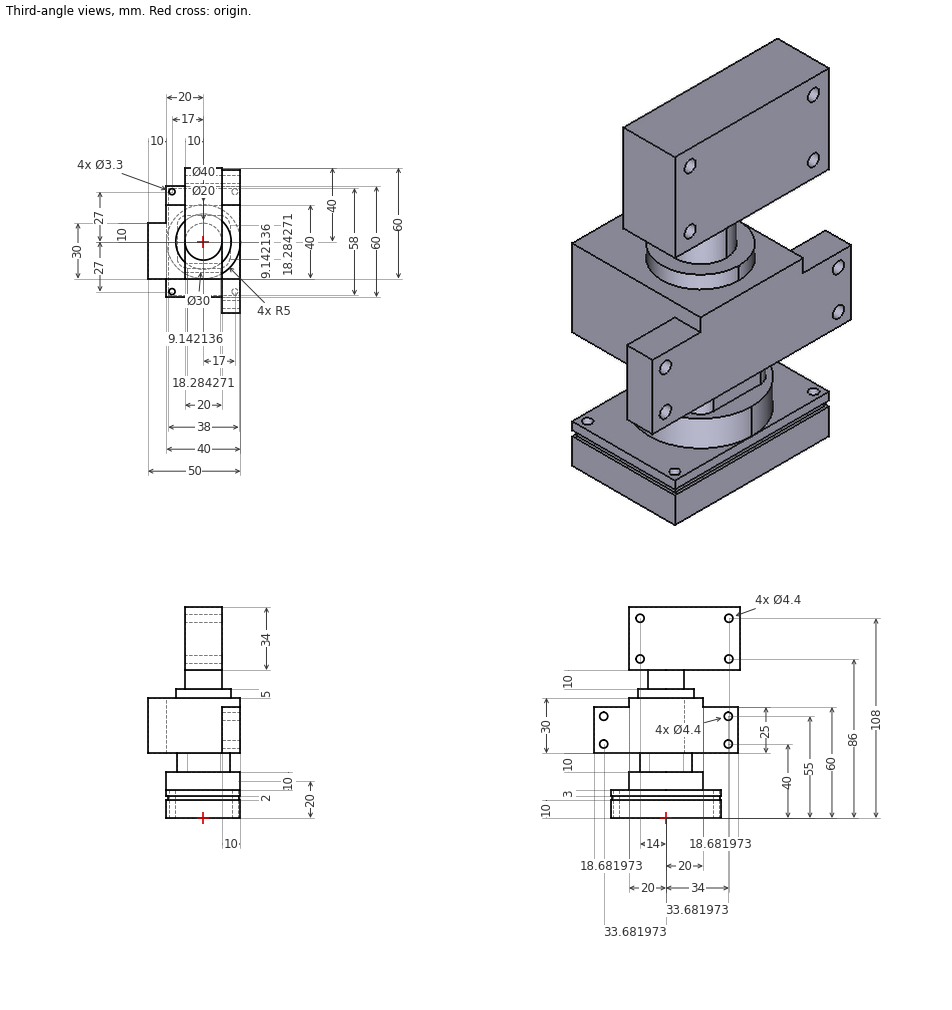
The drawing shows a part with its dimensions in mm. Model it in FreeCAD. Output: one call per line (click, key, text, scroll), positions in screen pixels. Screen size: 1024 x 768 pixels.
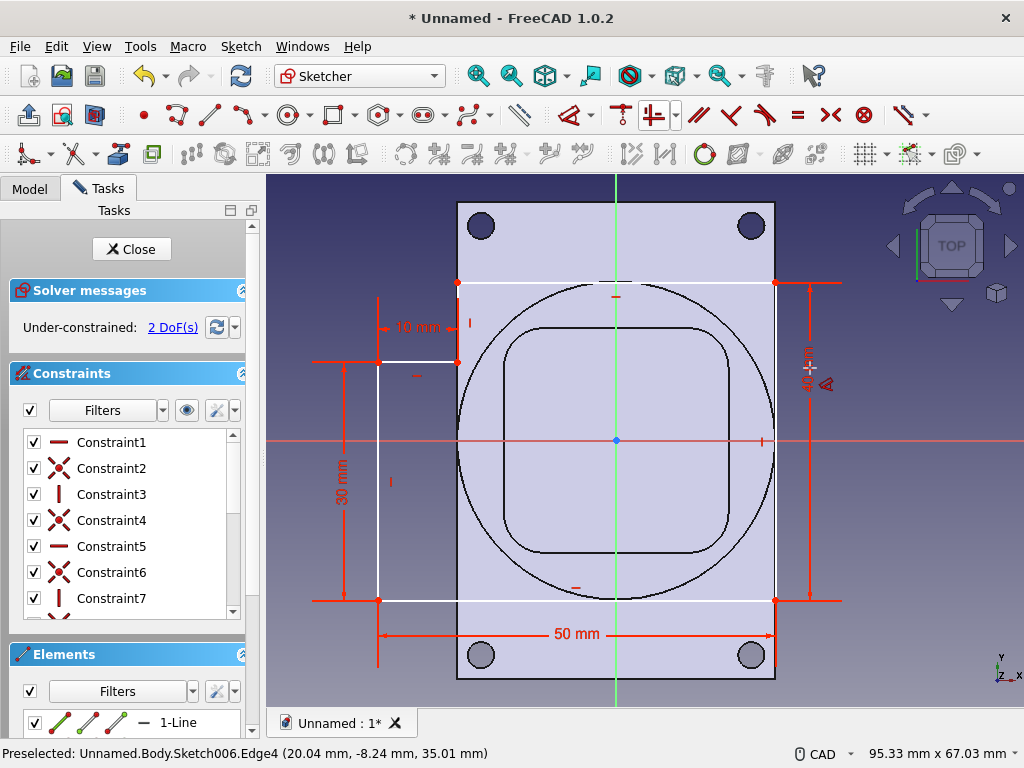
click(458, 362)
click(537, 328)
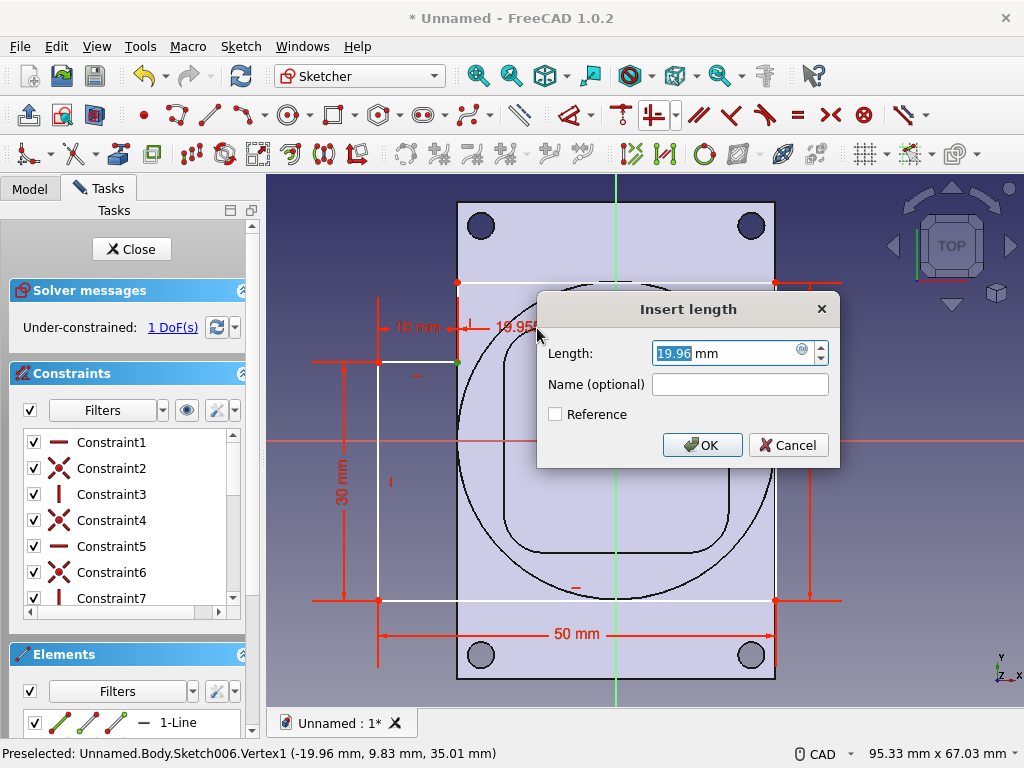
text(20)
key(Return)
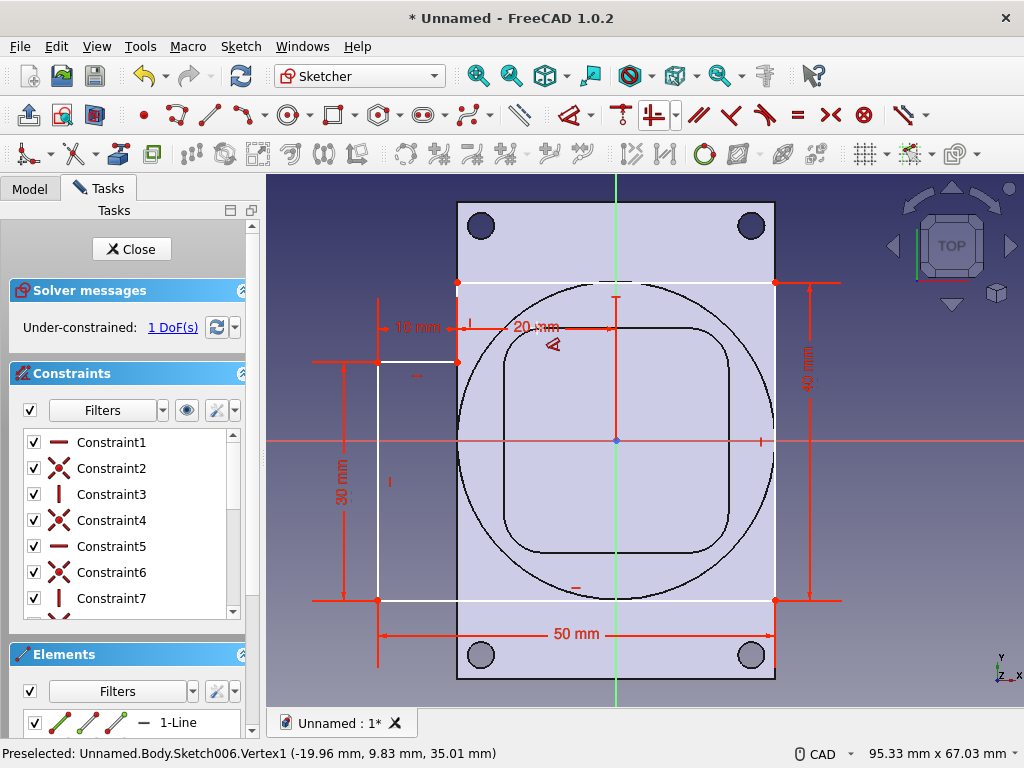
click(457, 362)
click(423, 401)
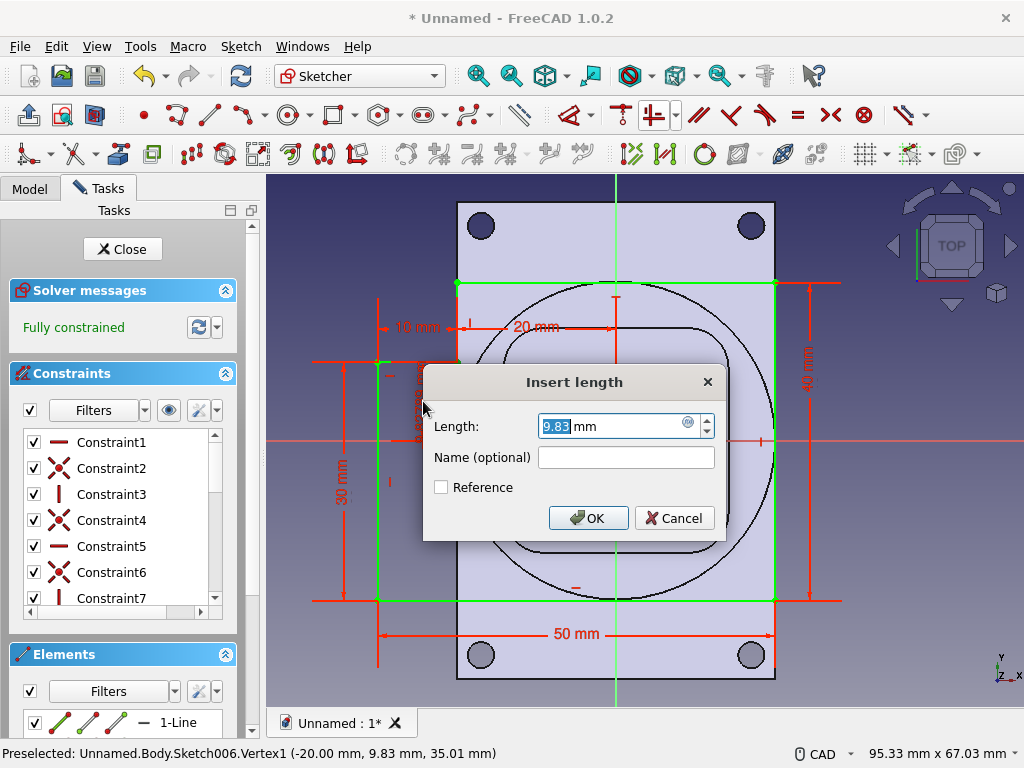
text(10)
key(Return)
key(Escape)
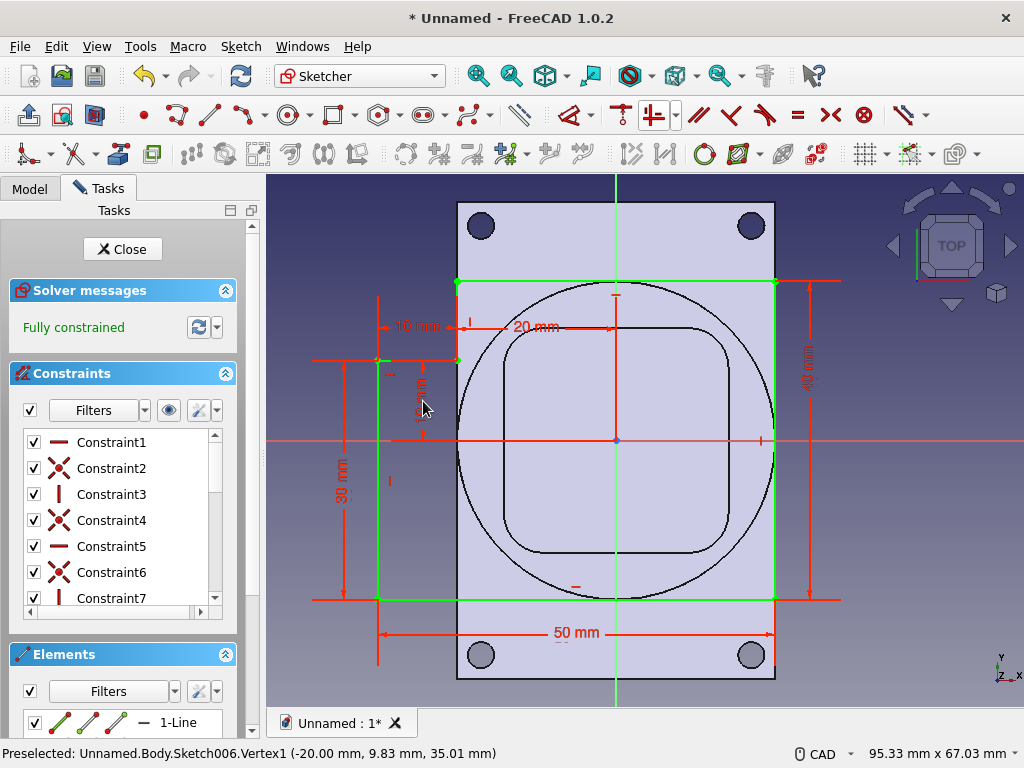
click(123, 249)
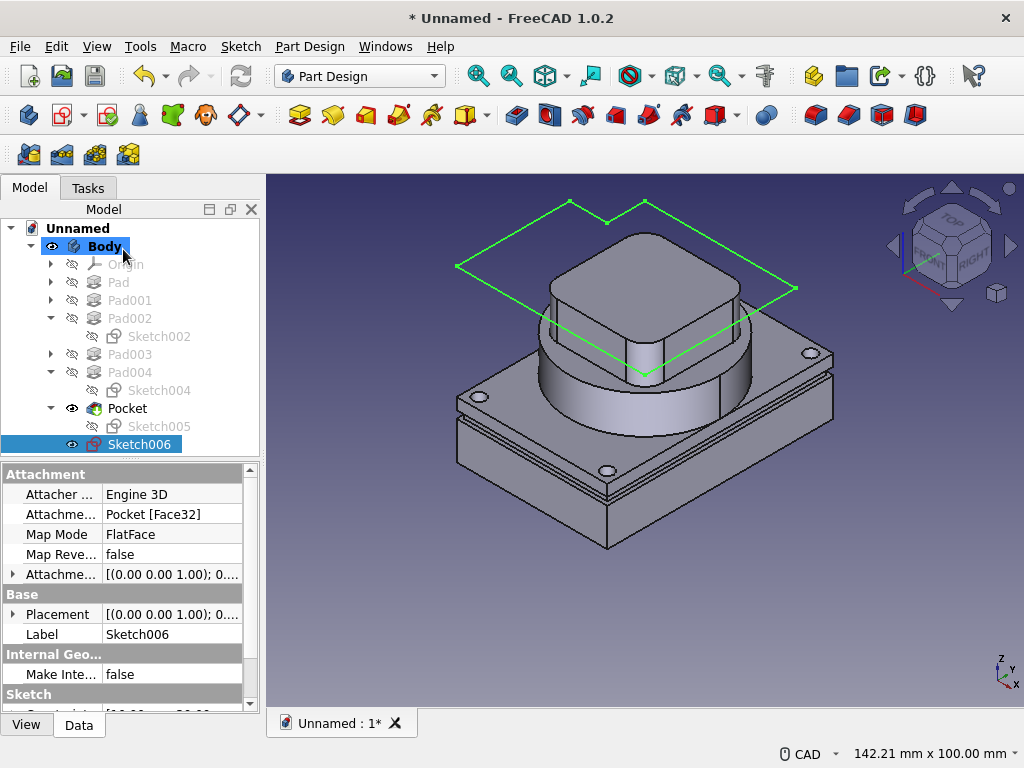
click(300, 116)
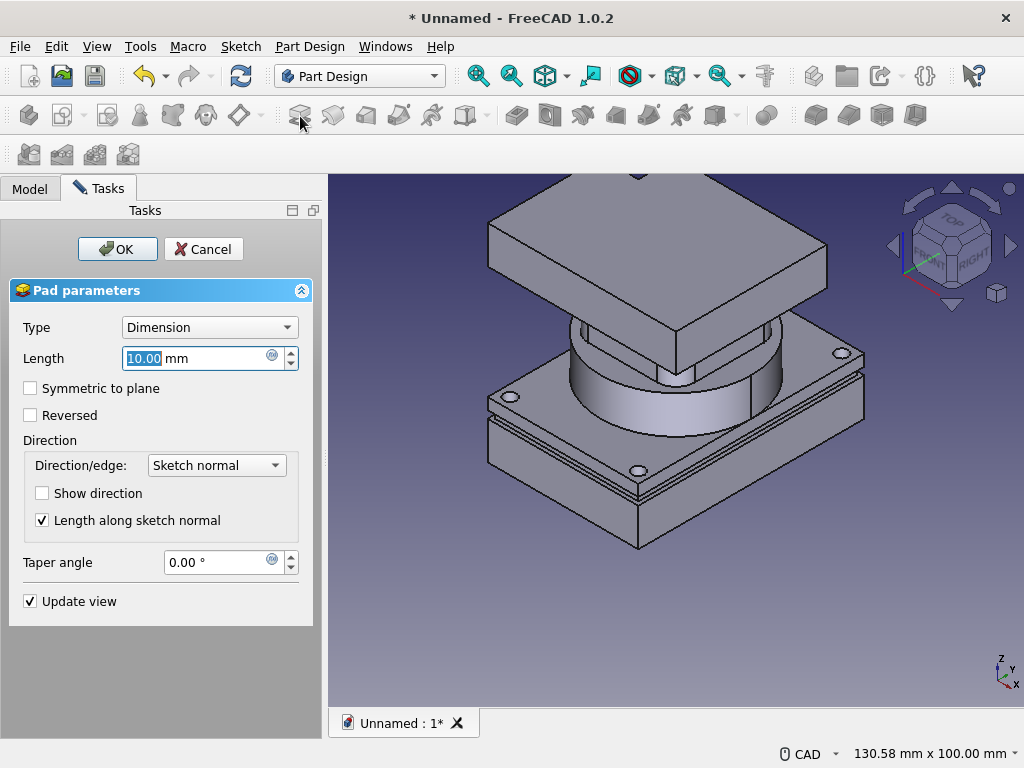
text(30)
key(Tab)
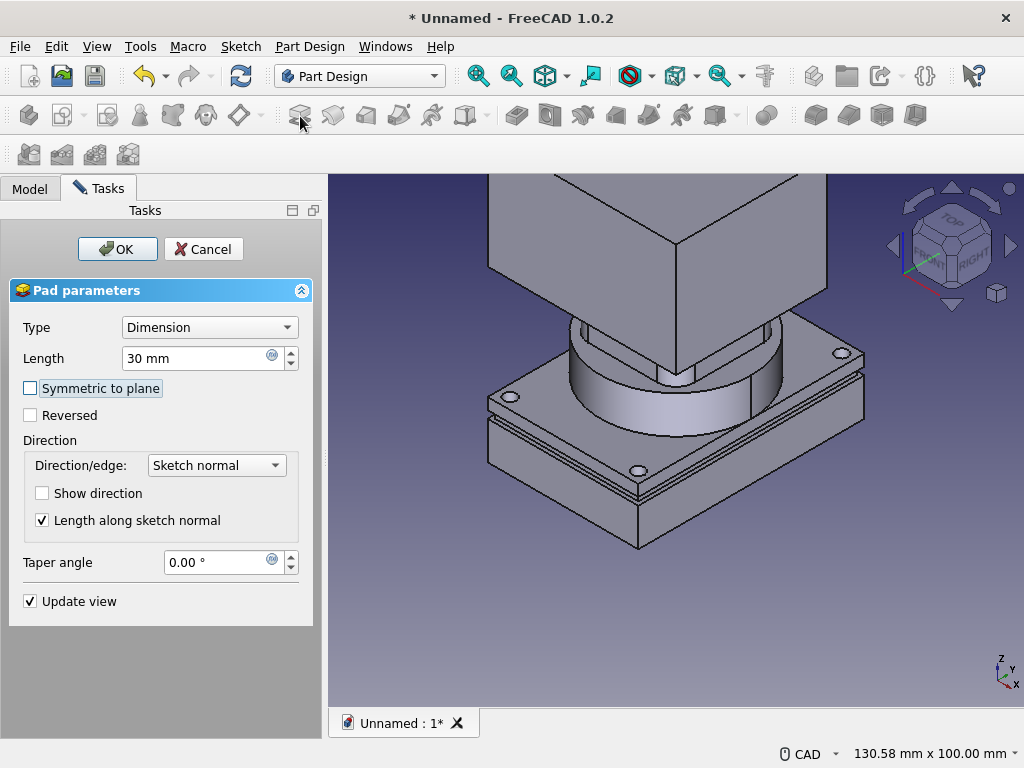
click(118, 249)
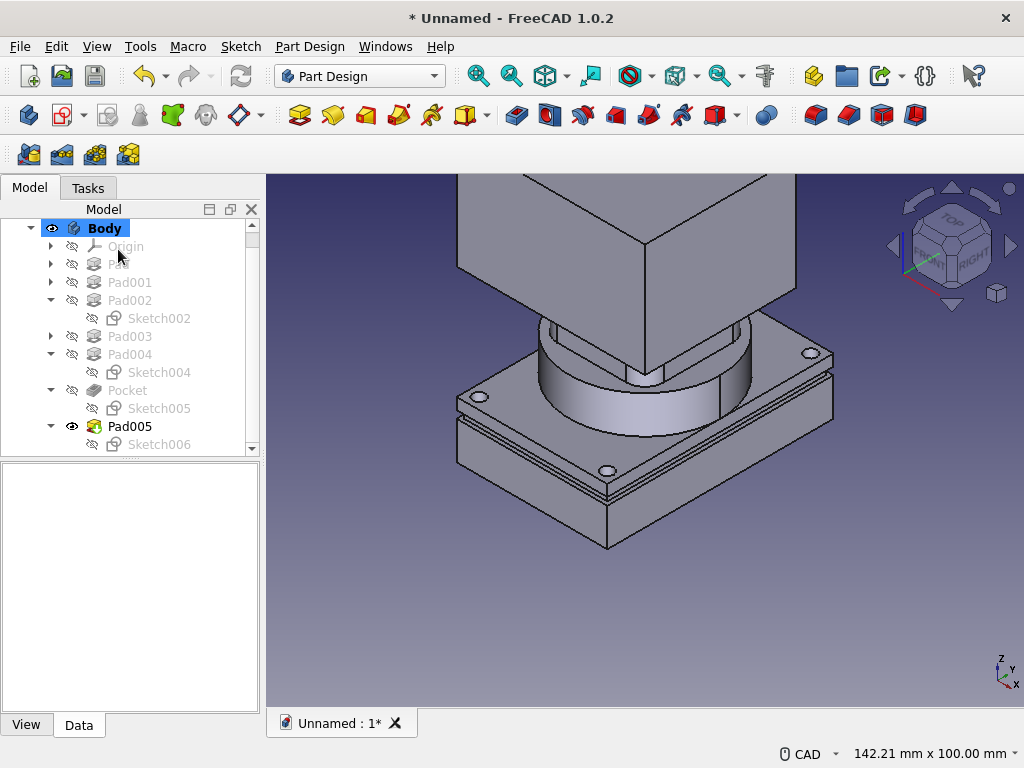
key(v)
key(f)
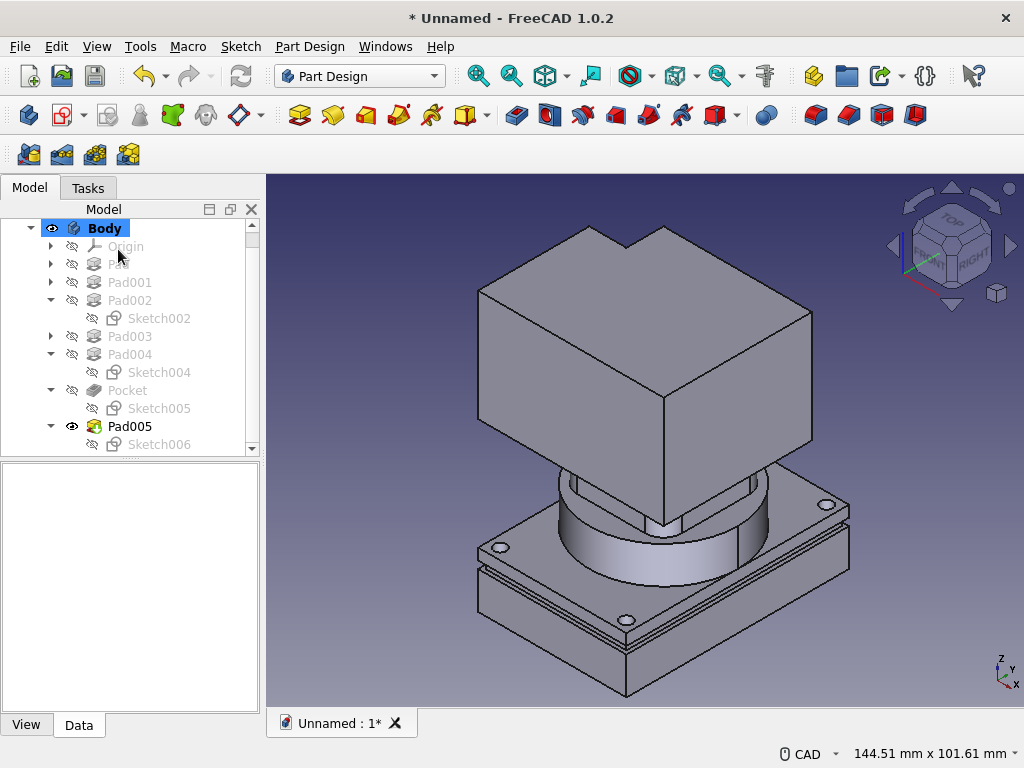
click(645, 300)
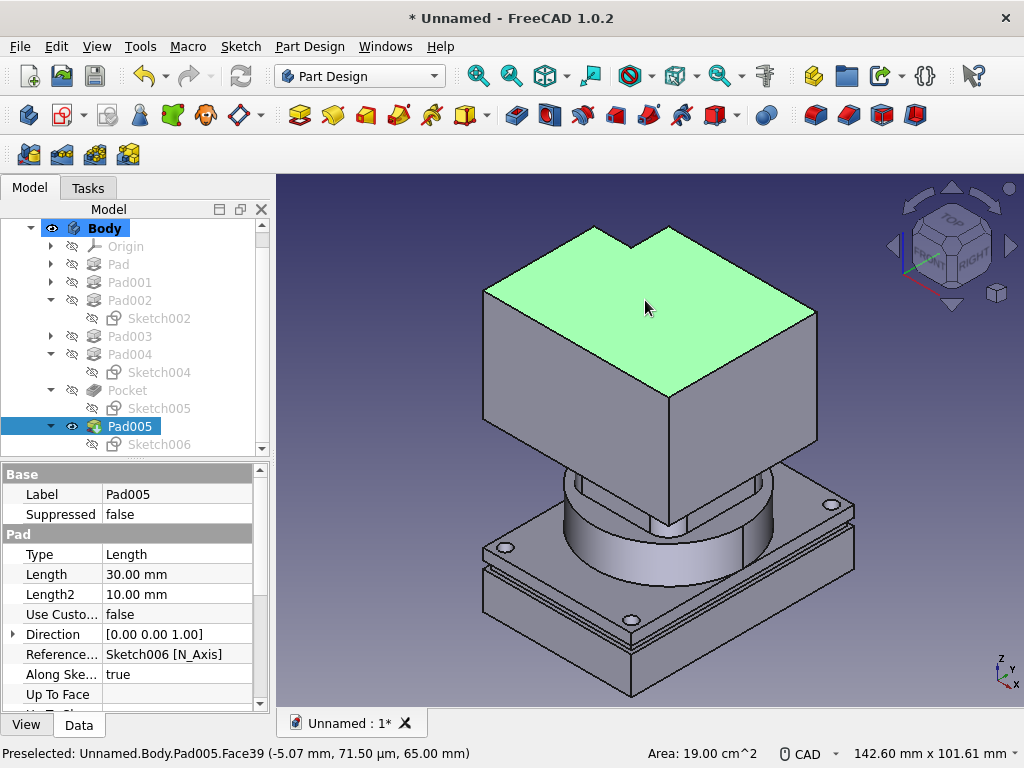
click(62, 116)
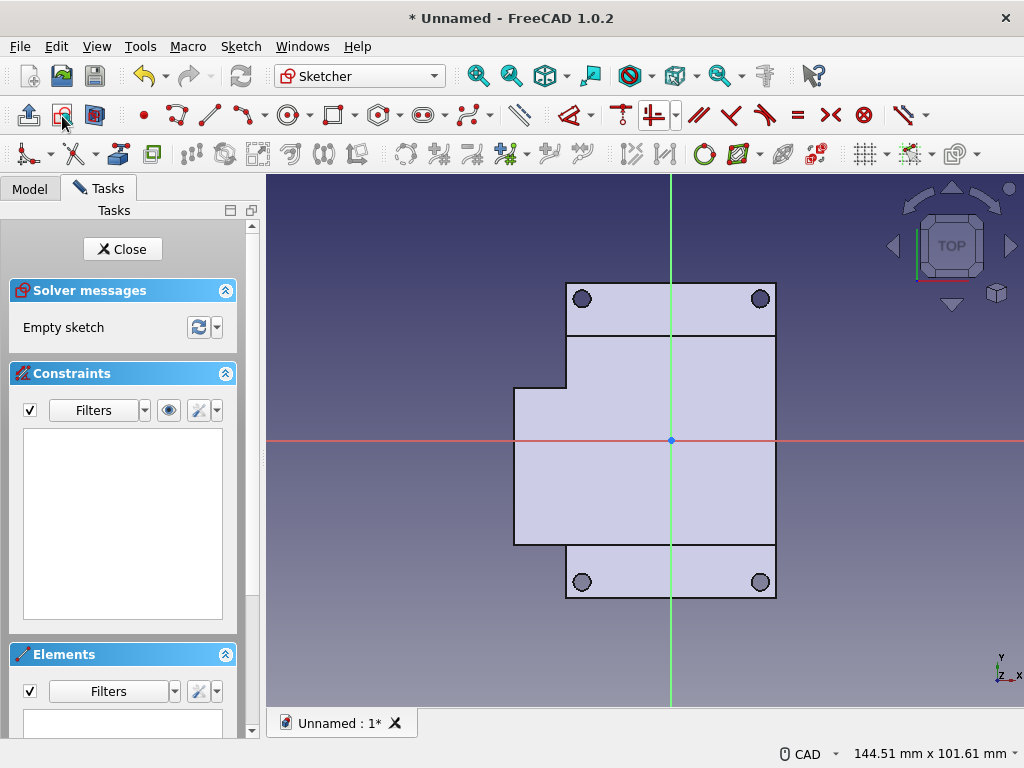
scroll(749, 440, up, 4)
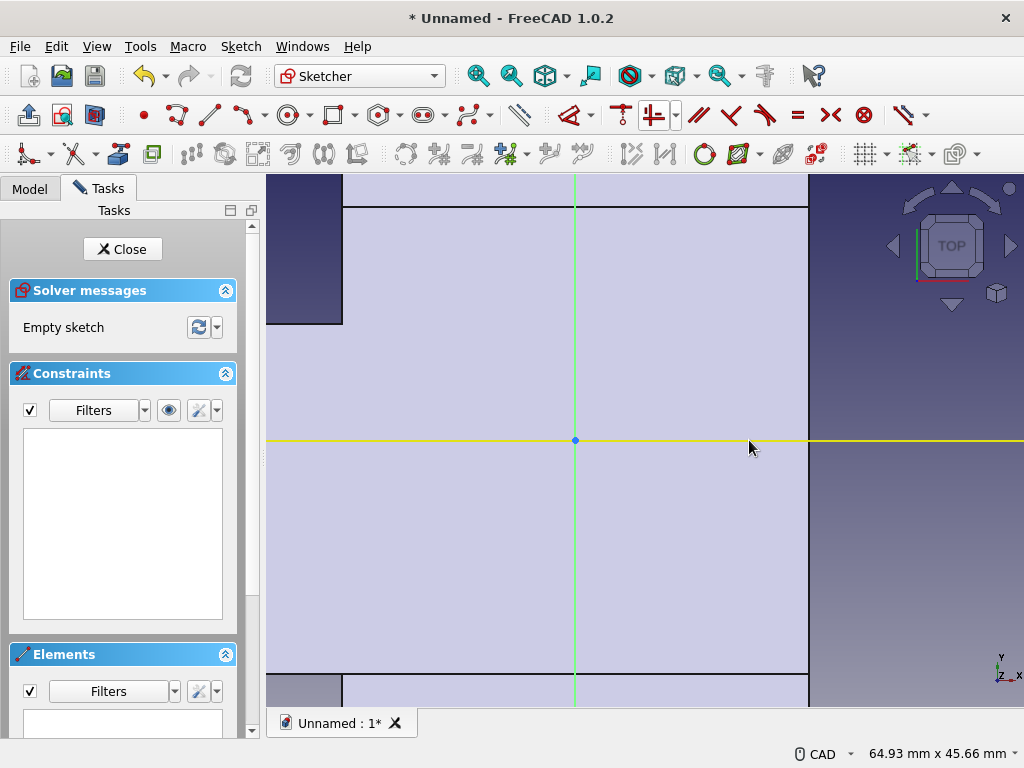
click(288, 116)